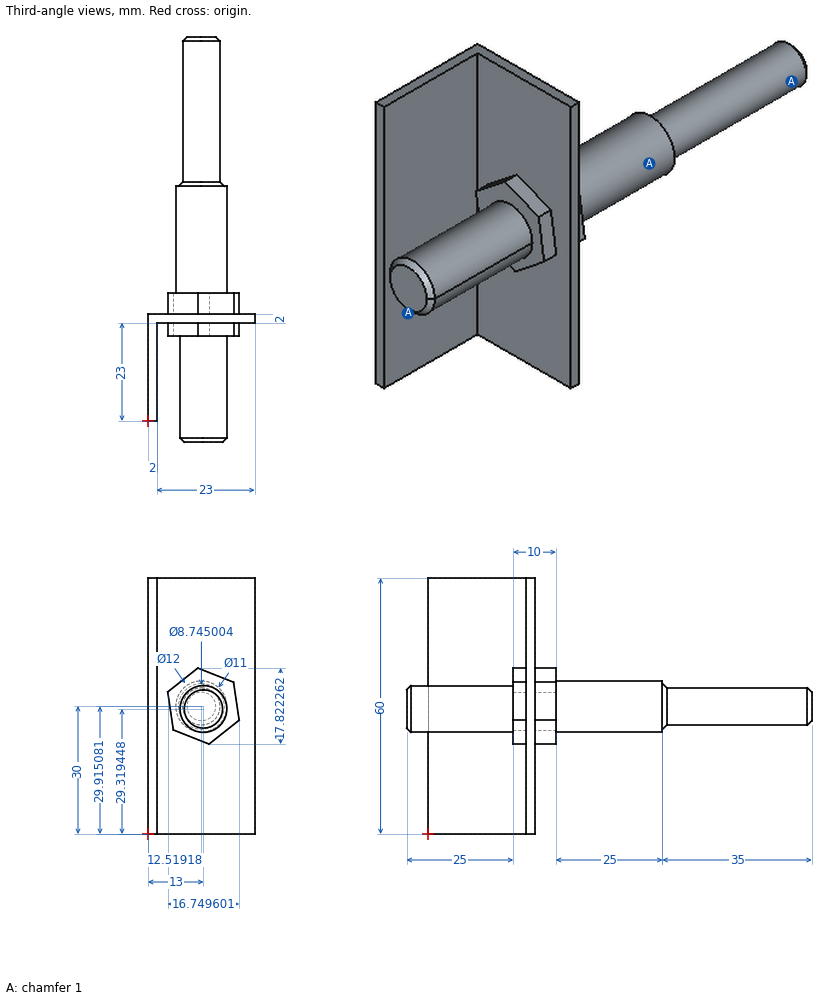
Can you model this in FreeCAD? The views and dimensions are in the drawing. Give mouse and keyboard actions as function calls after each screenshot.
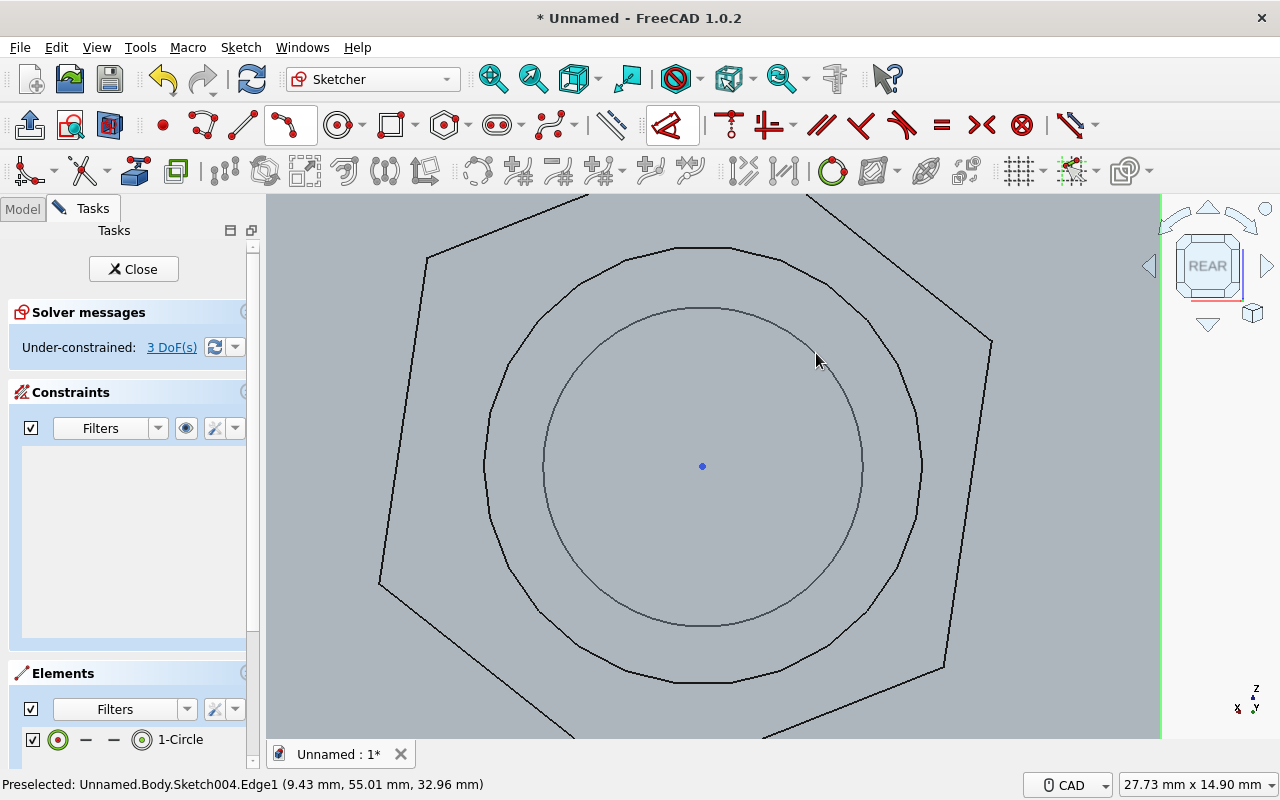
click(816, 354)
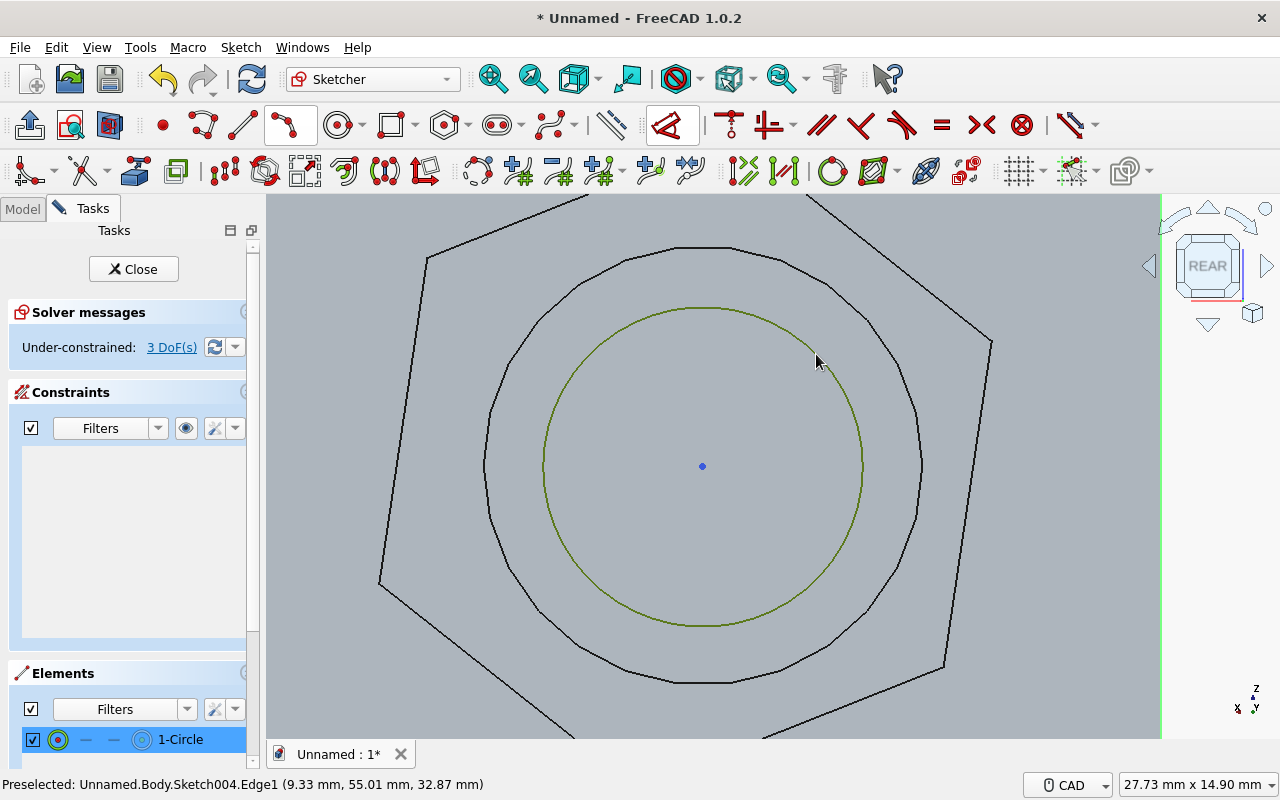
key(k)
key(o)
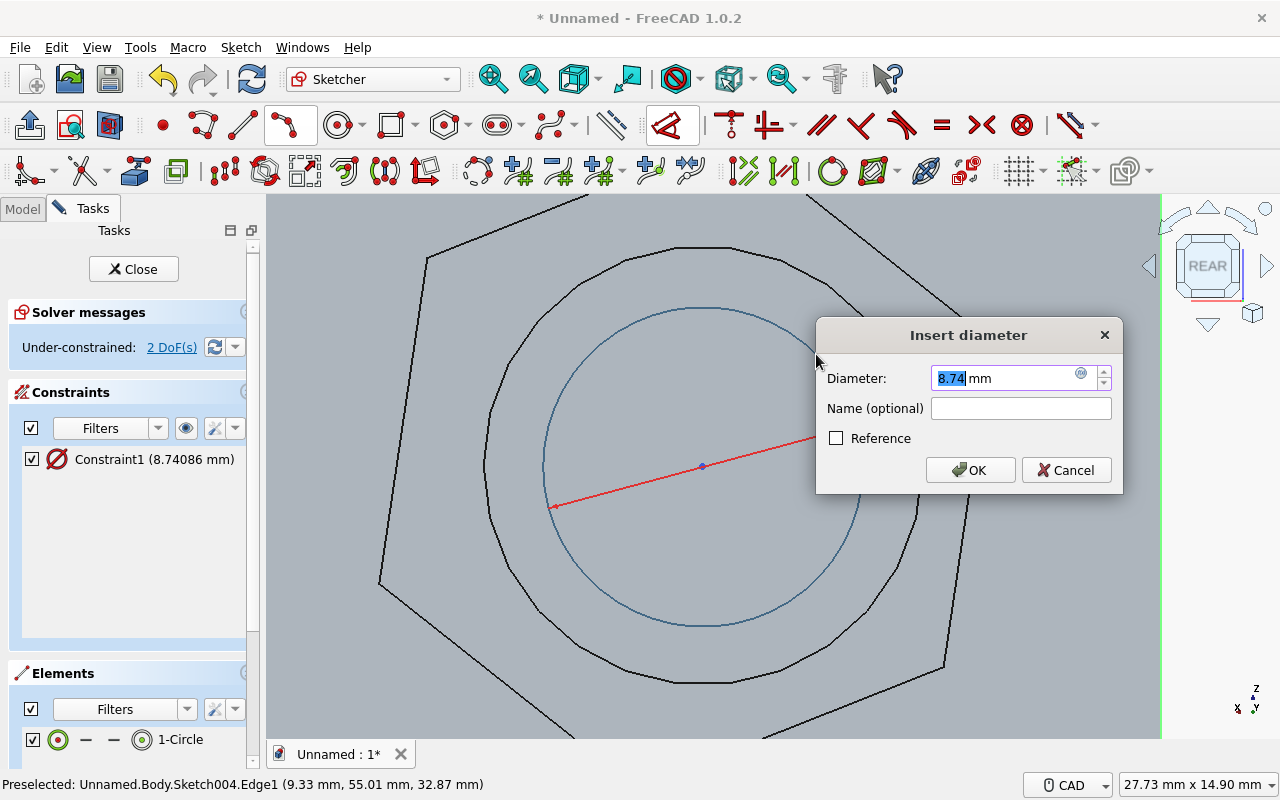
text(8.745004)
key(Return)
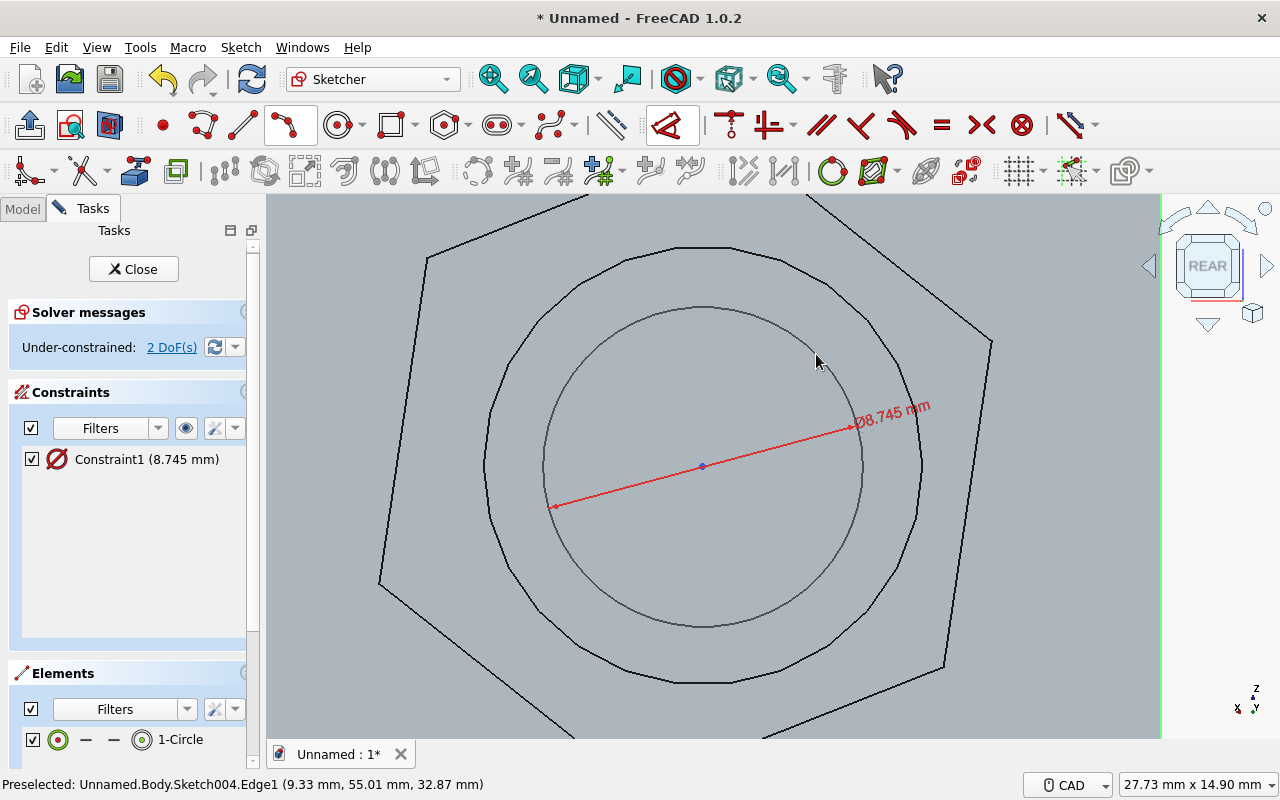
click(703, 467)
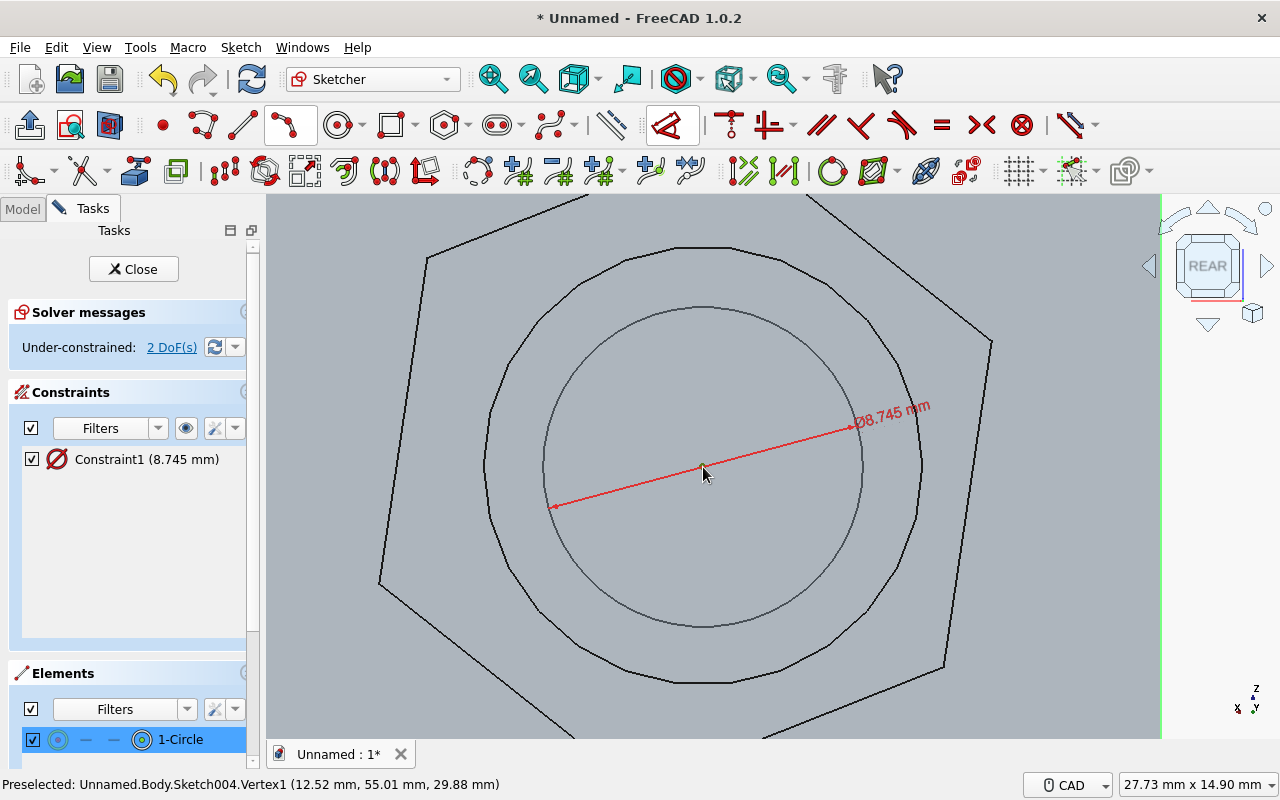
click(694, 126)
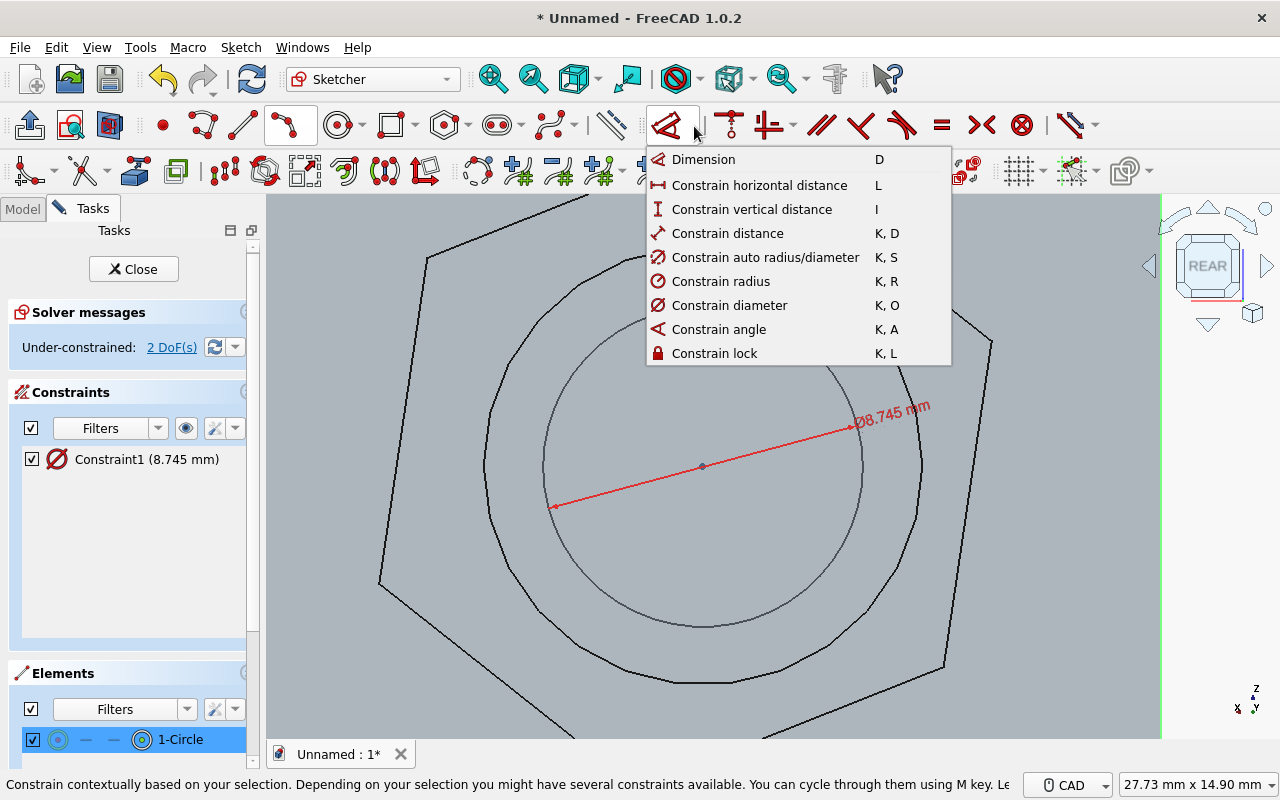
click(799, 185)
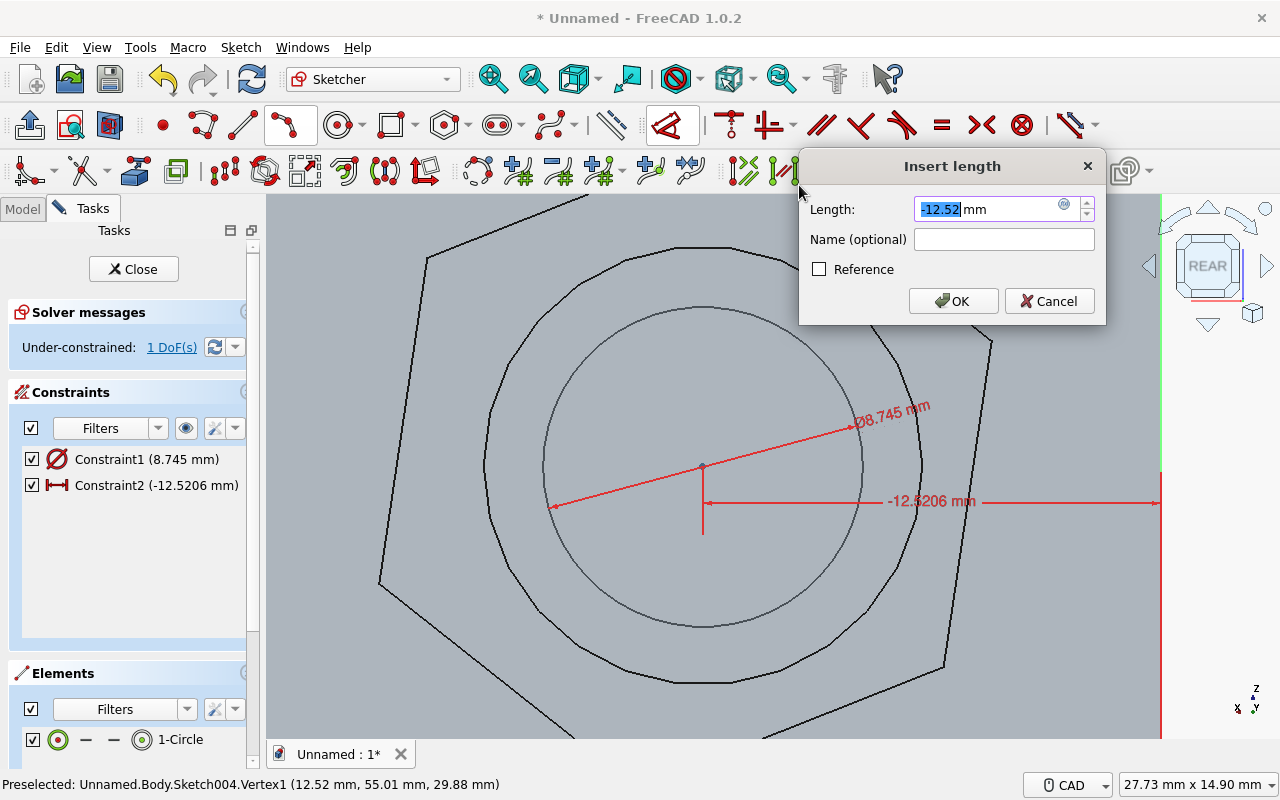
text(-12.51918)
key(Return)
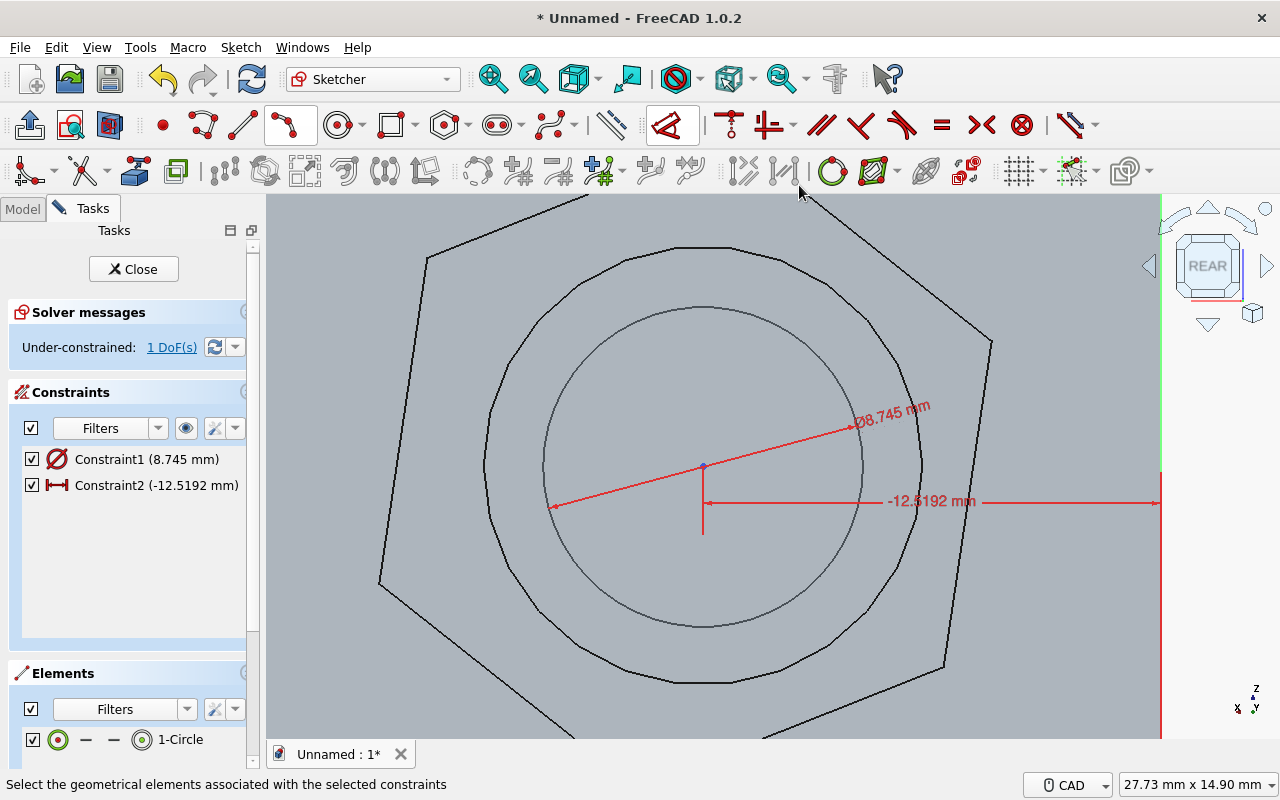
click(703, 467)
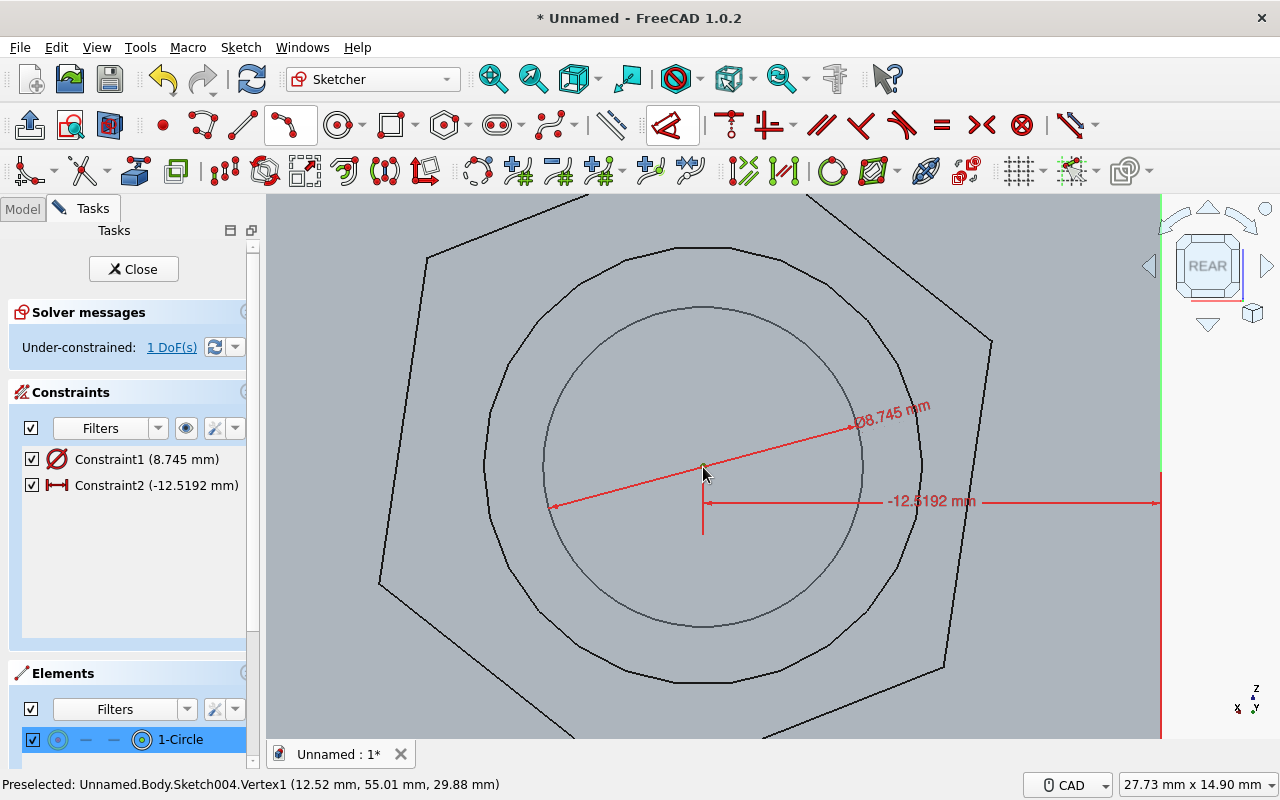
click(694, 126)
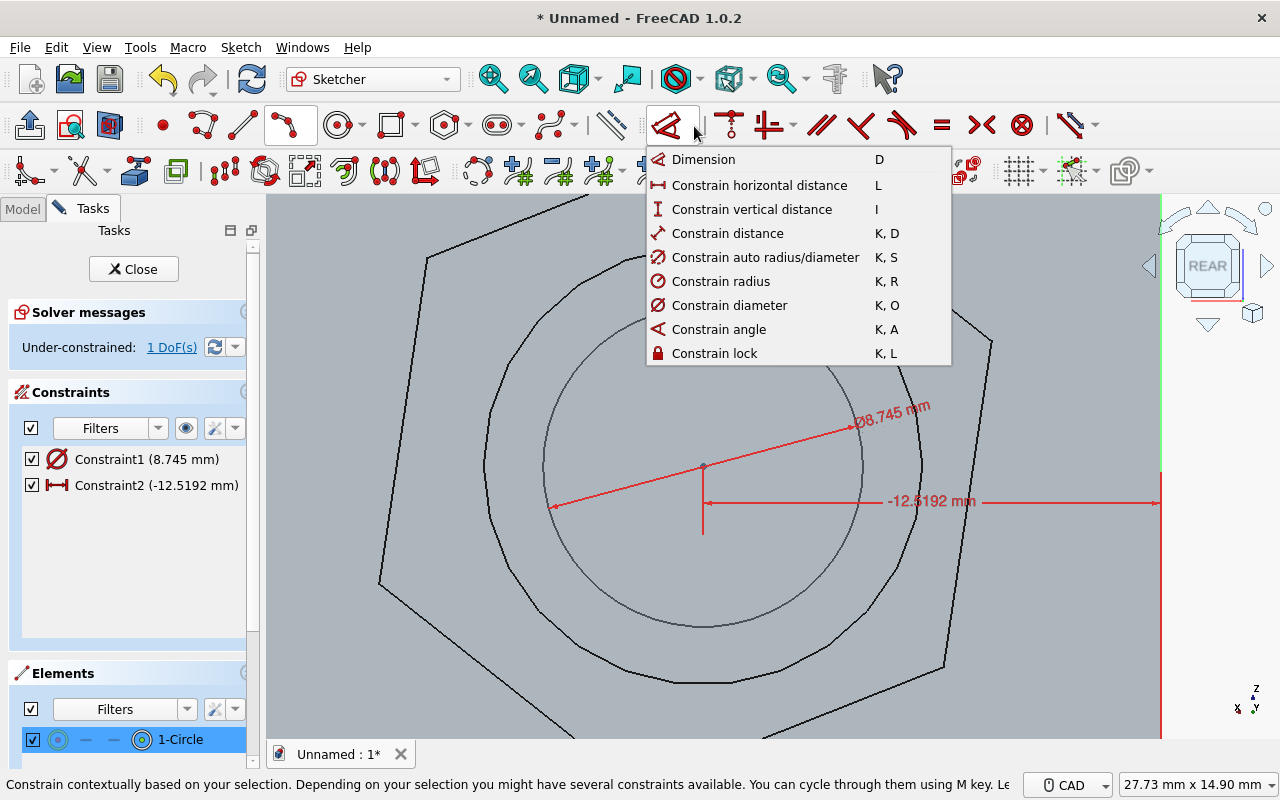
click(799, 209)